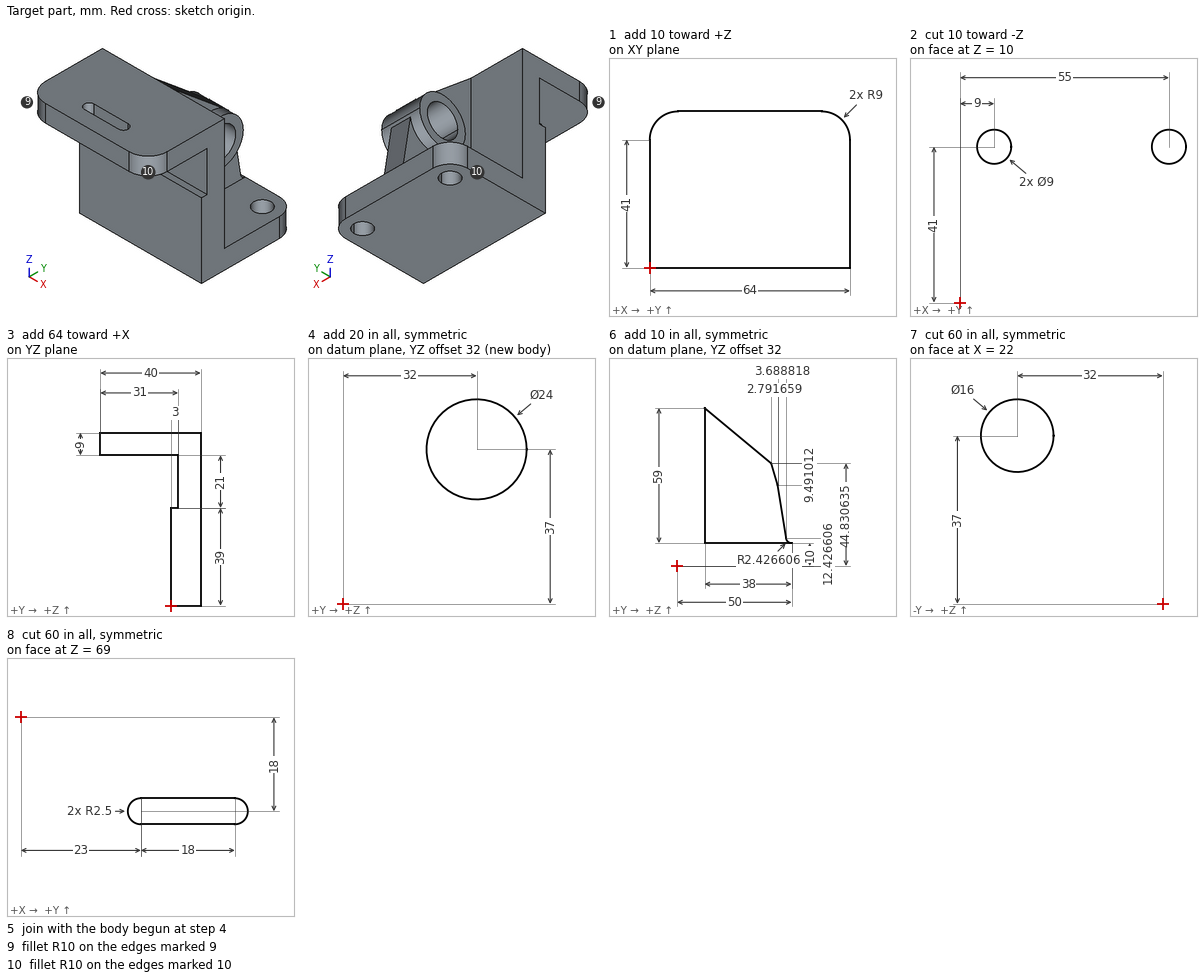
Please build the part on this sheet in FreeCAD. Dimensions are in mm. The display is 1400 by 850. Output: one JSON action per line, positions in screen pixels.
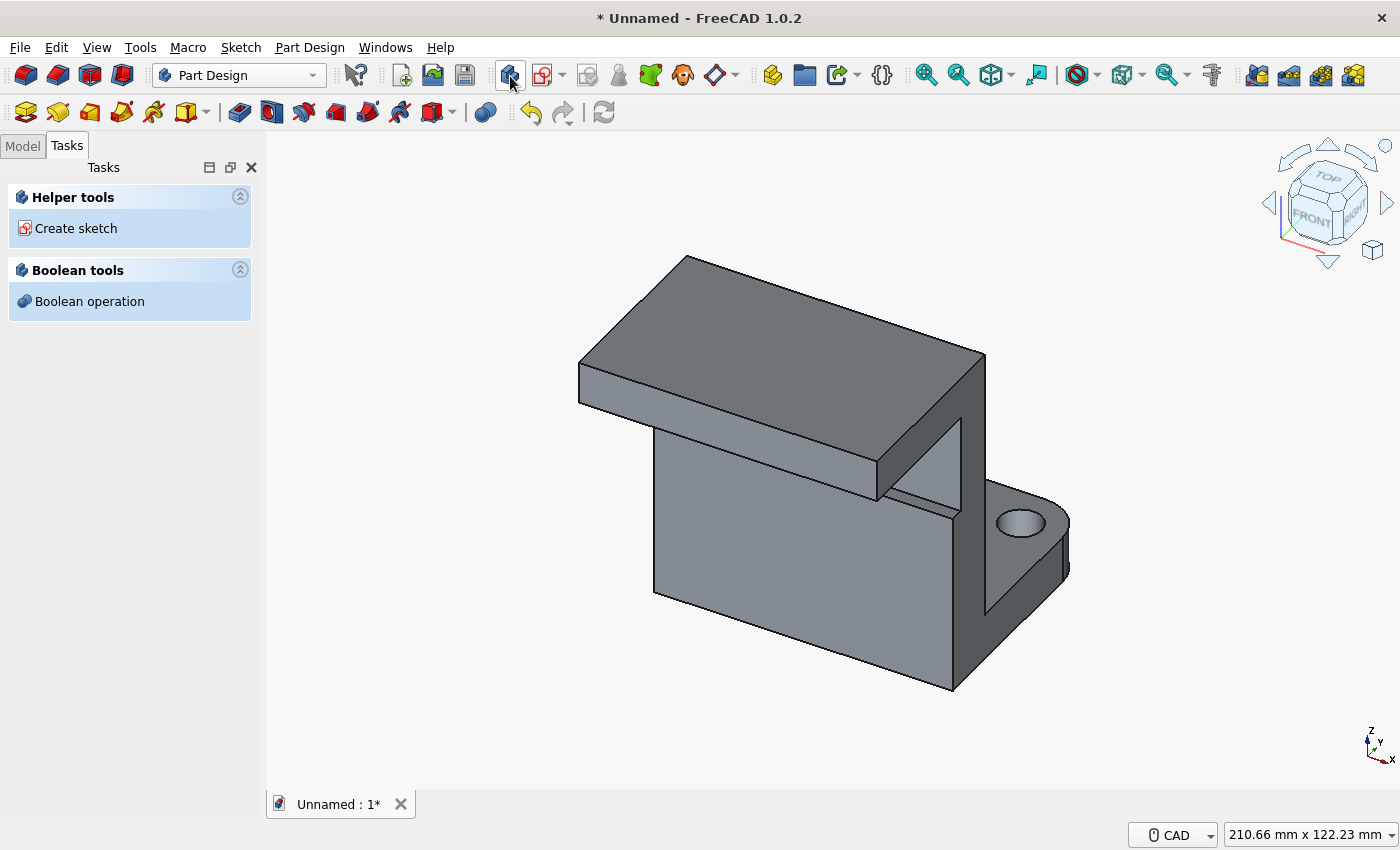
{"action": "left_click", "coordinate": [23, 145]}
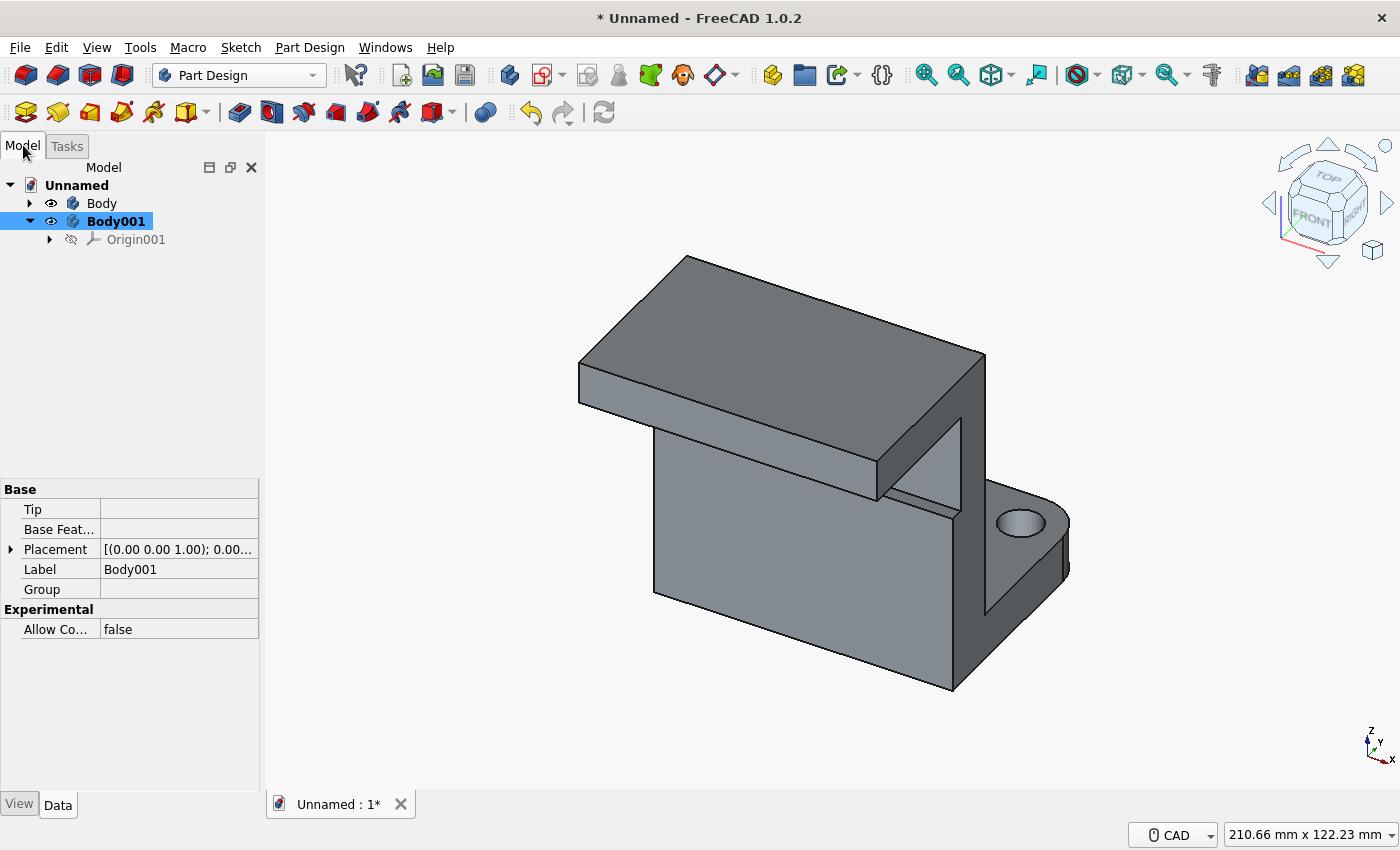
{"action": "left_click", "coordinate": [50, 239]}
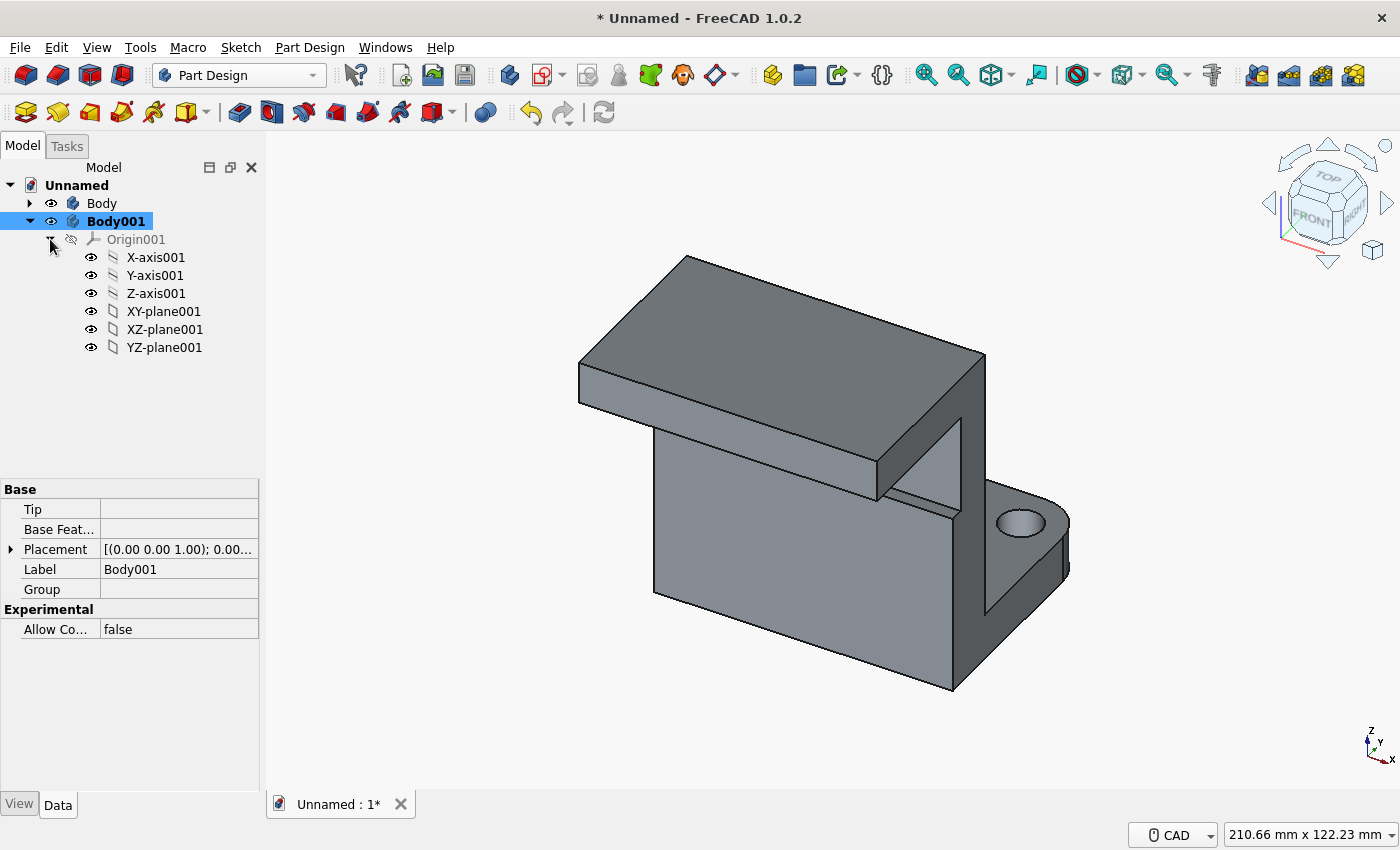
{"action": "left_click", "coordinate": [136, 347]}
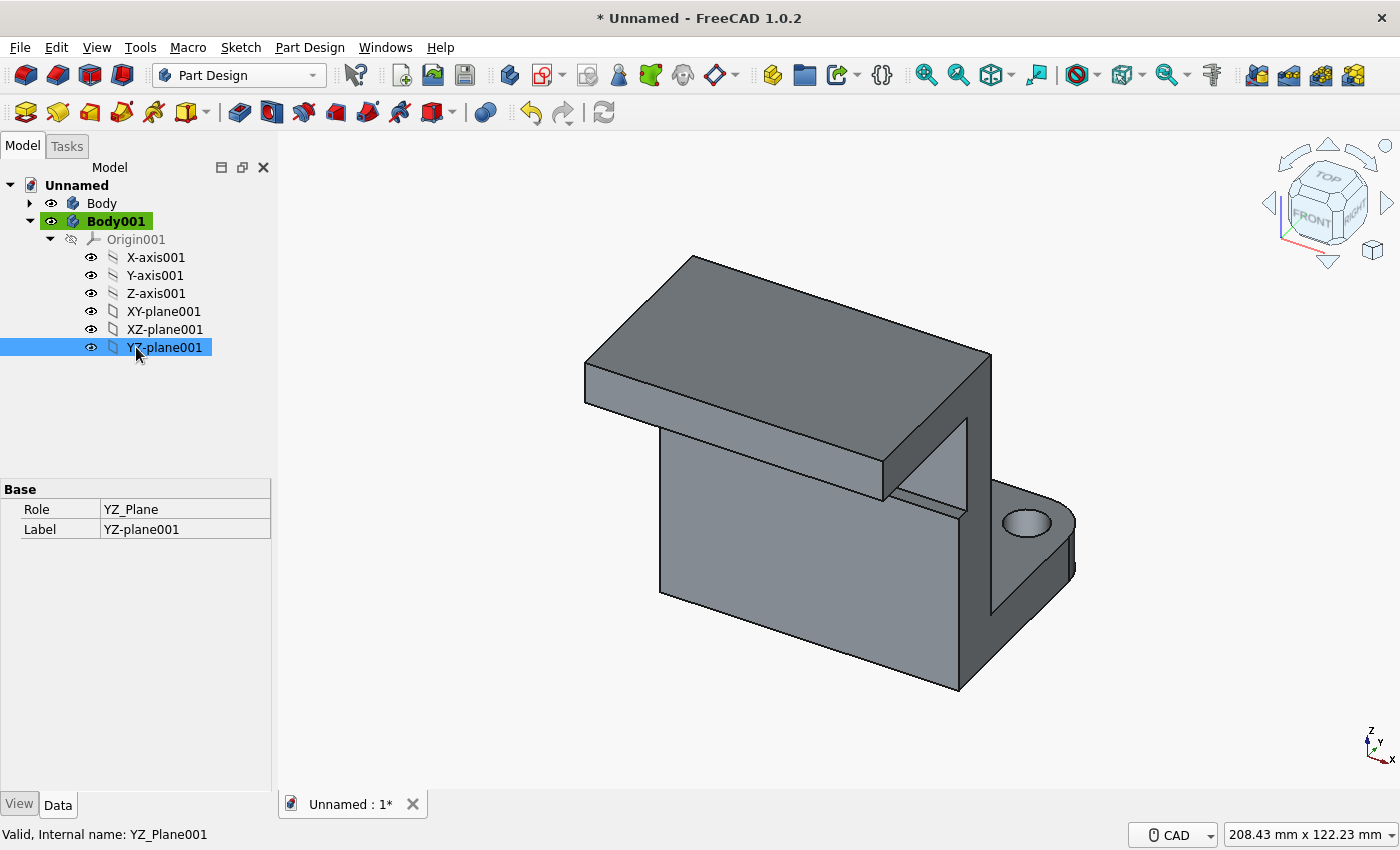
{"action": "left_click", "coordinate": [716, 76]}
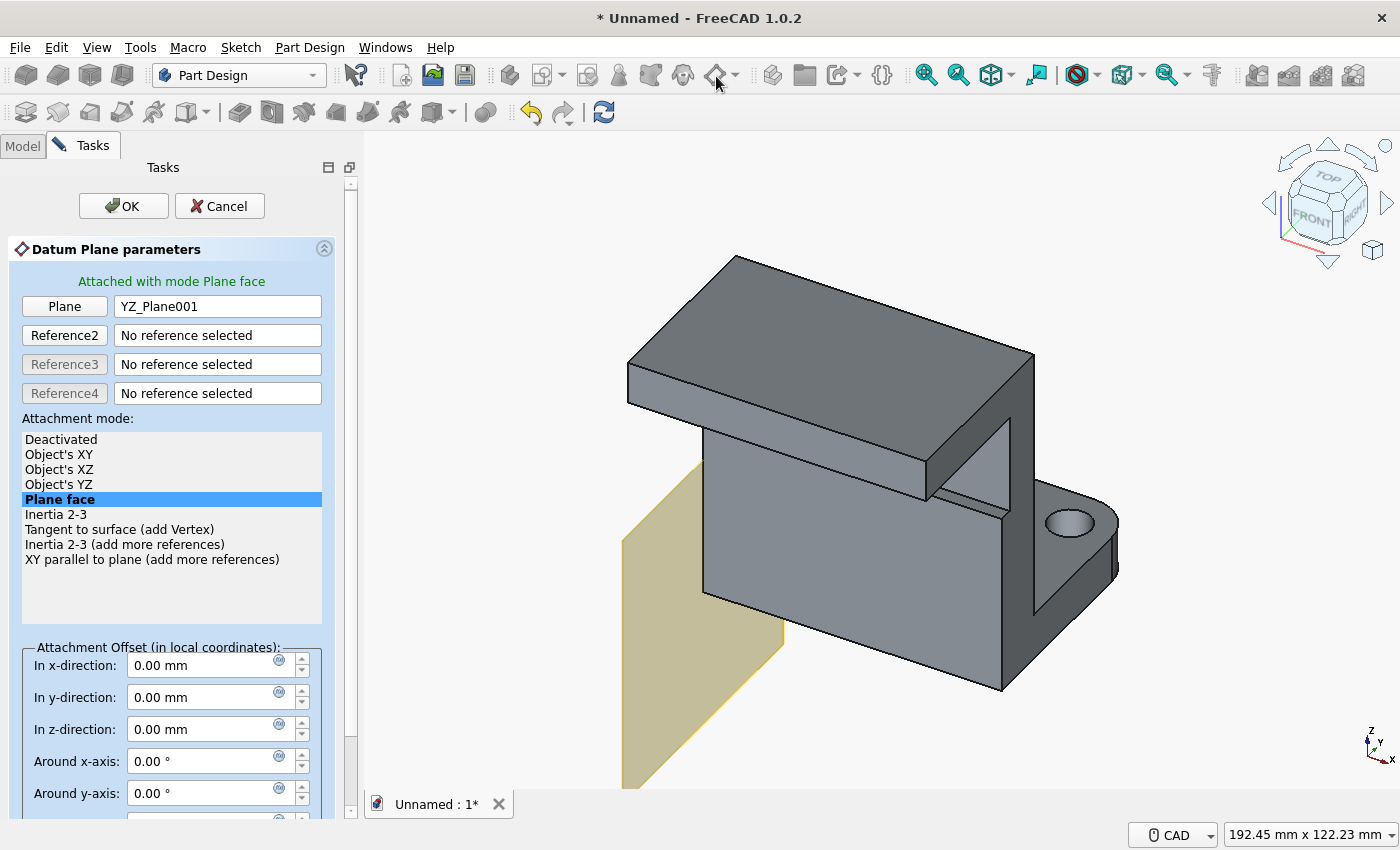
{"action": "triple_click", "coordinate": [210, 729]}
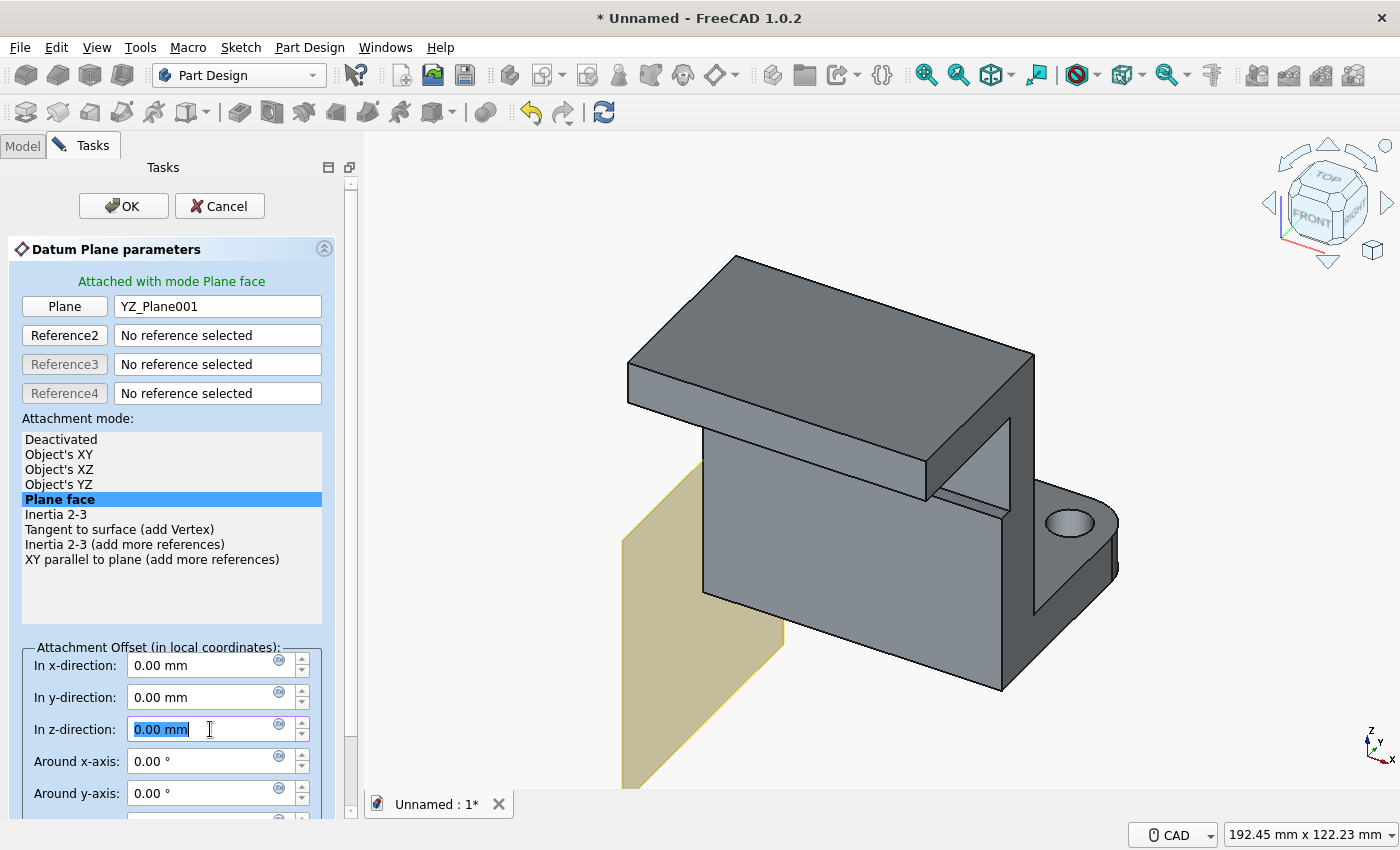
{"action": "type", "text": "32"}
{"action": "key", "text": "Tab"}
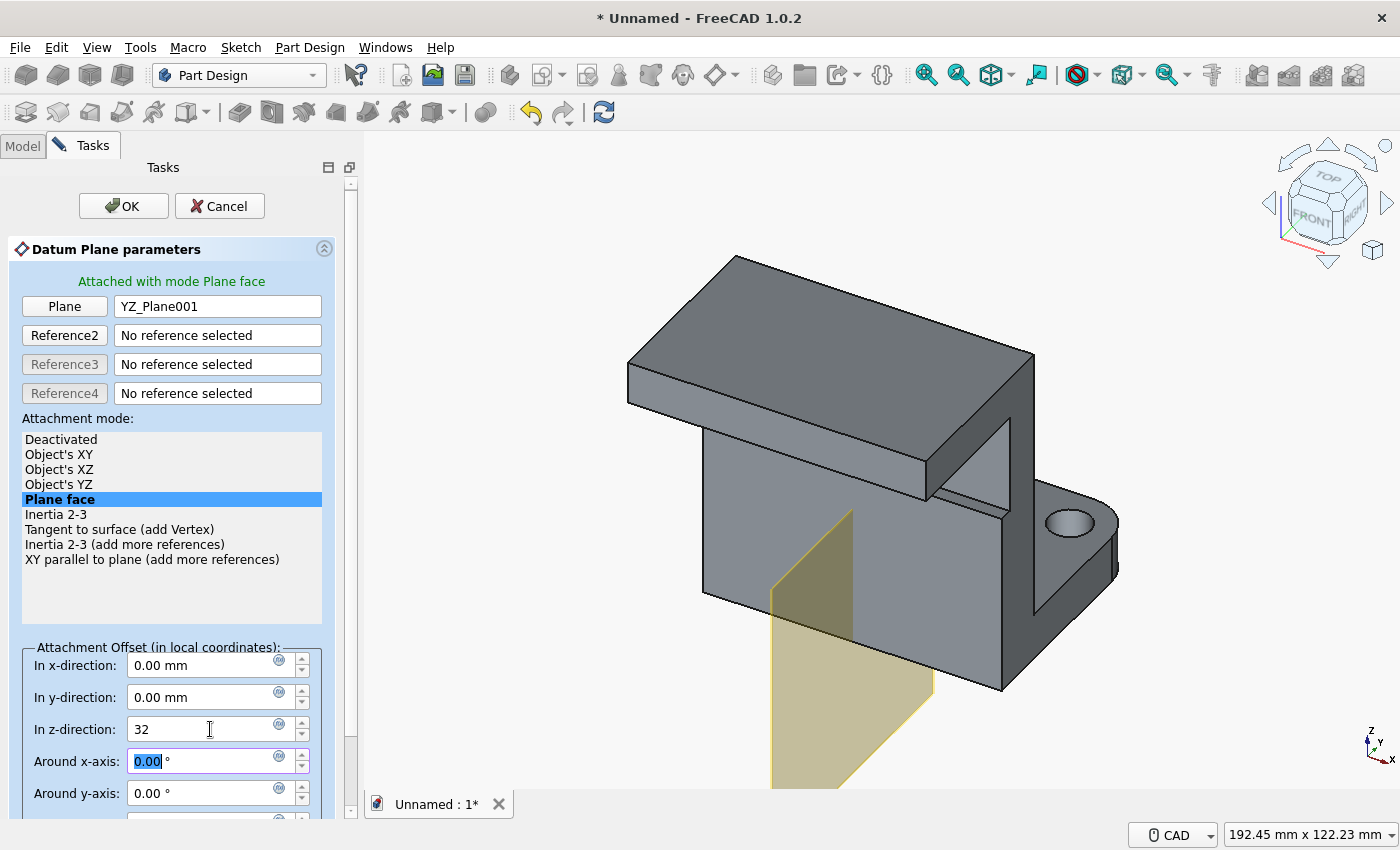
{"action": "left_click", "coordinate": [124, 206]}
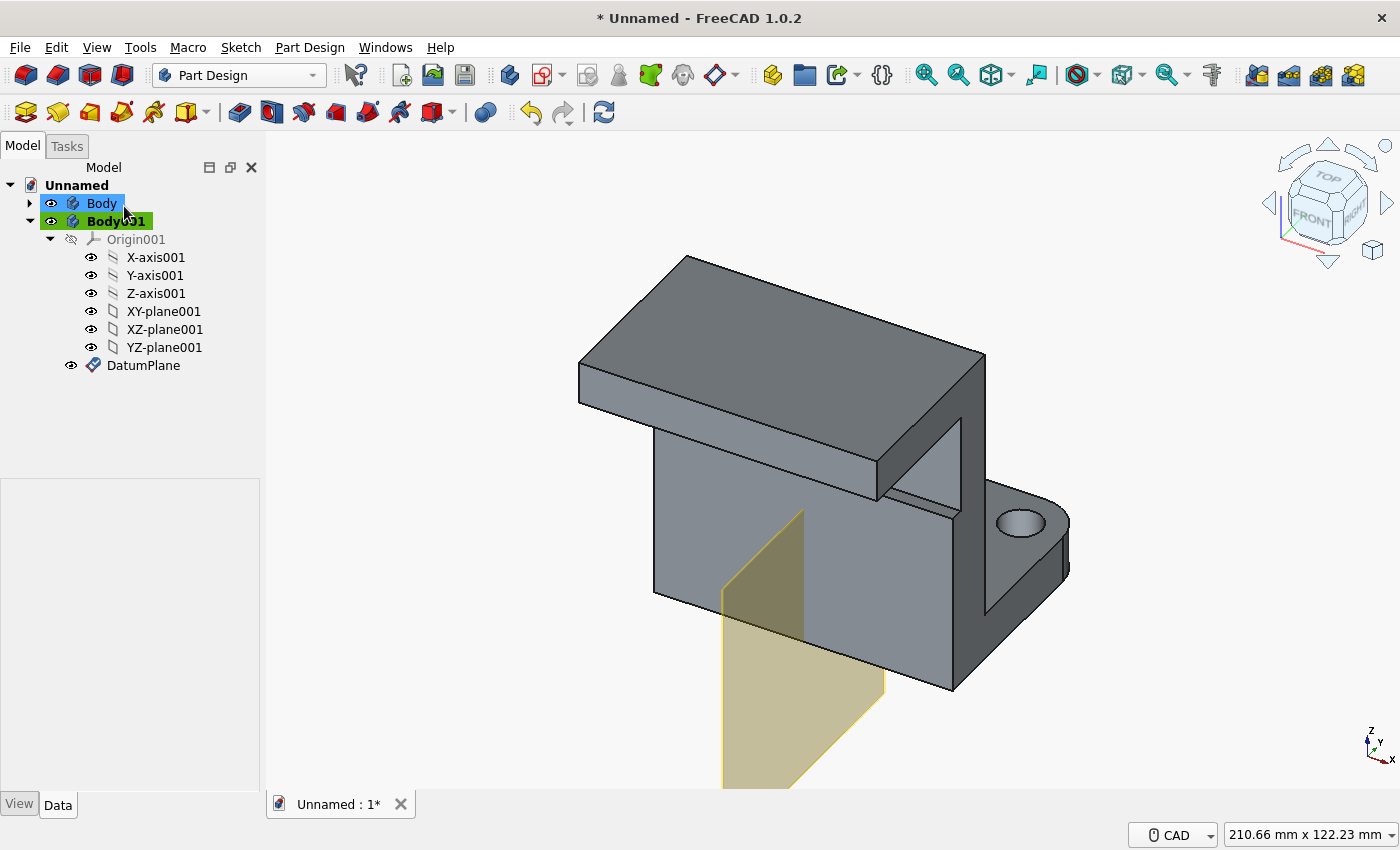
{"action": "left_click", "coordinate": [116, 365]}